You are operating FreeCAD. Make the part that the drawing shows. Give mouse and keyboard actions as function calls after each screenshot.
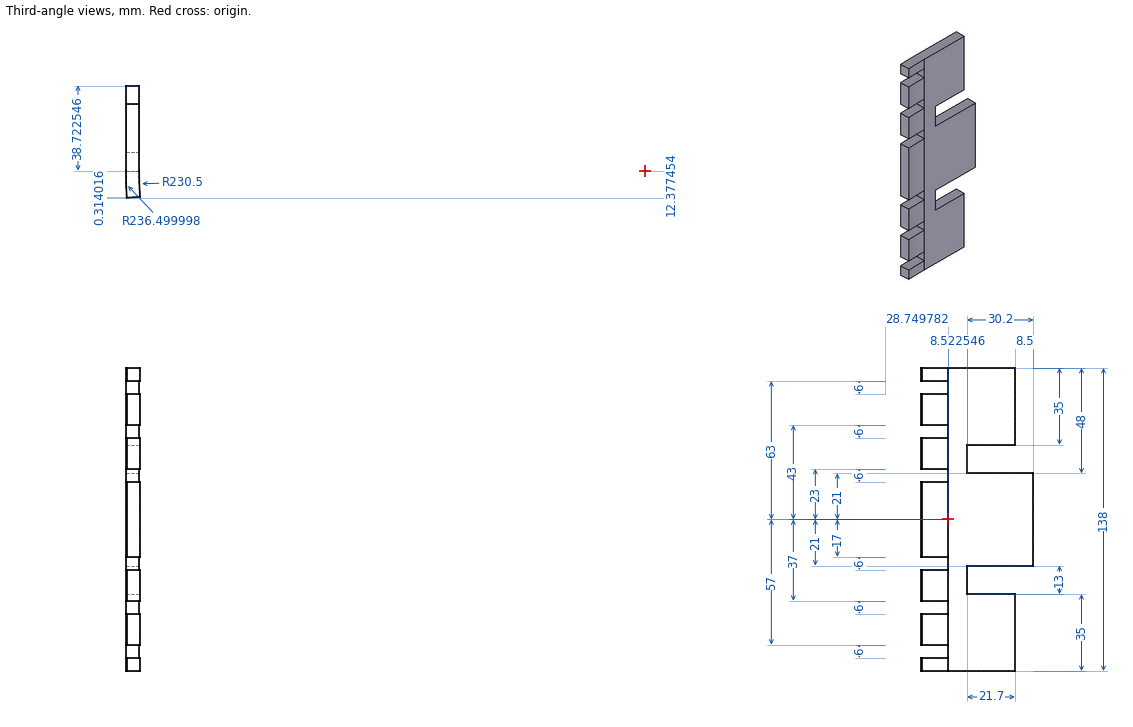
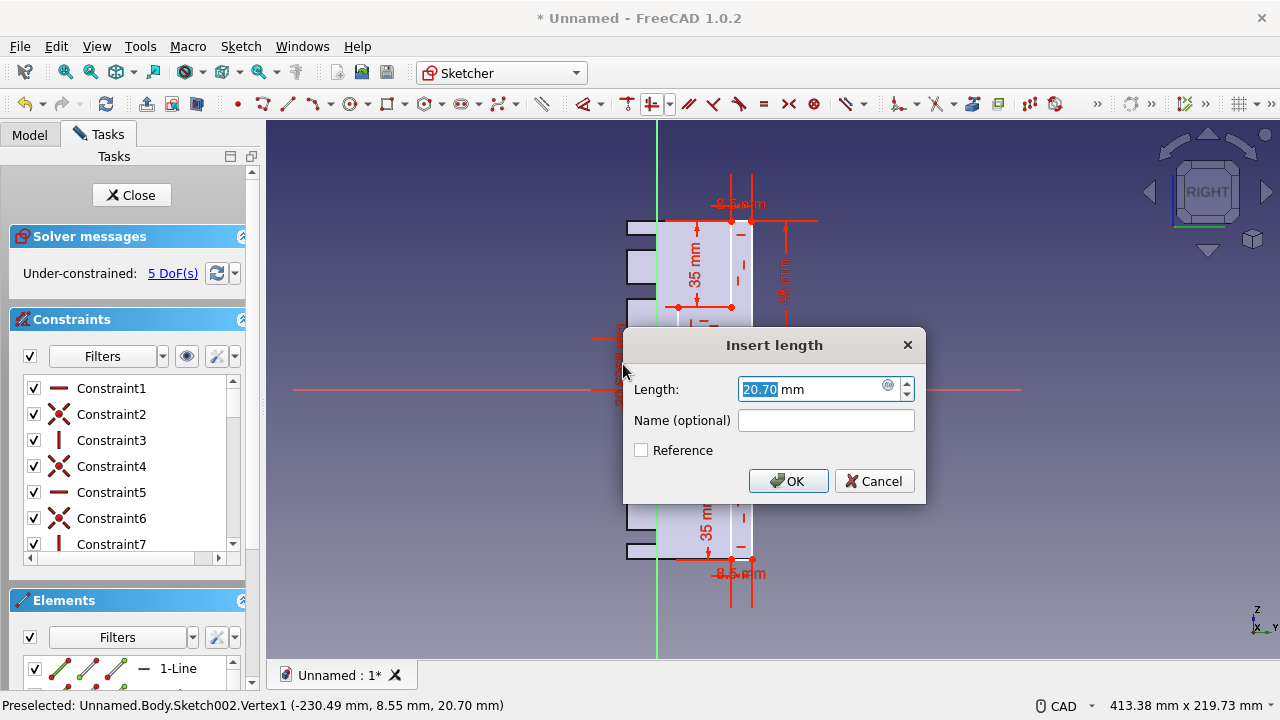
text(21)
key(Return)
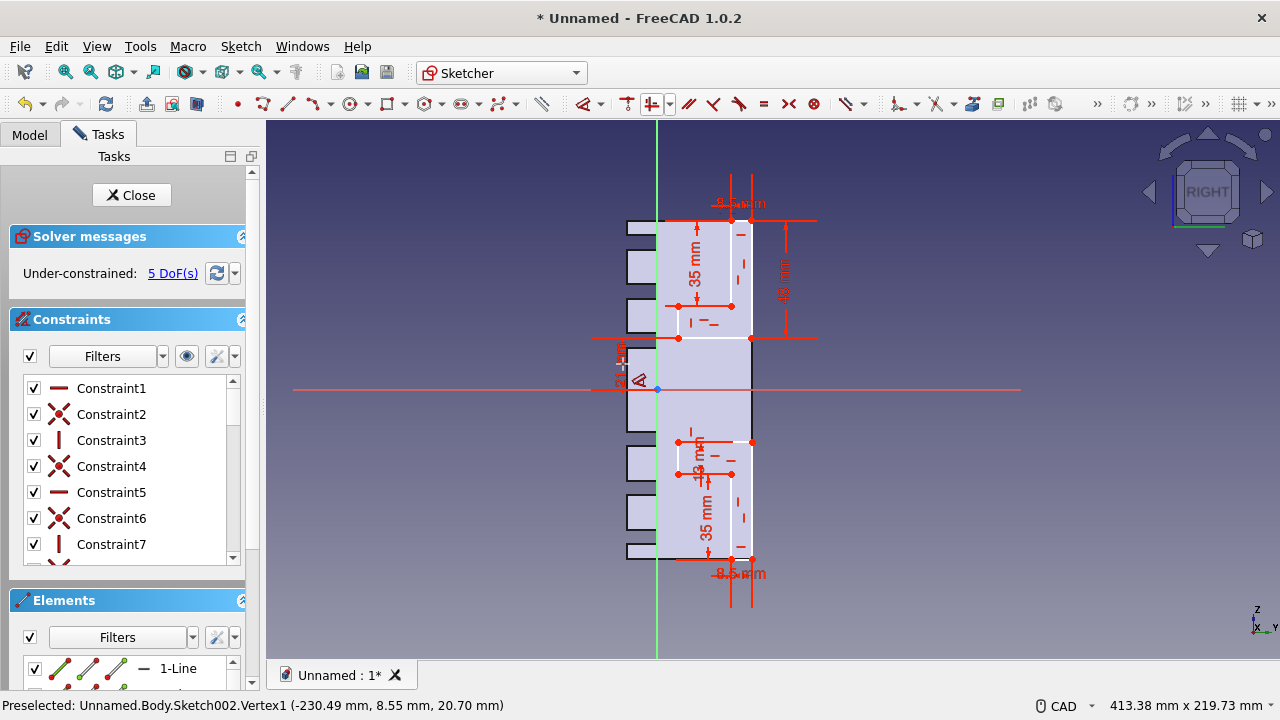
click(678, 442)
click(623, 416)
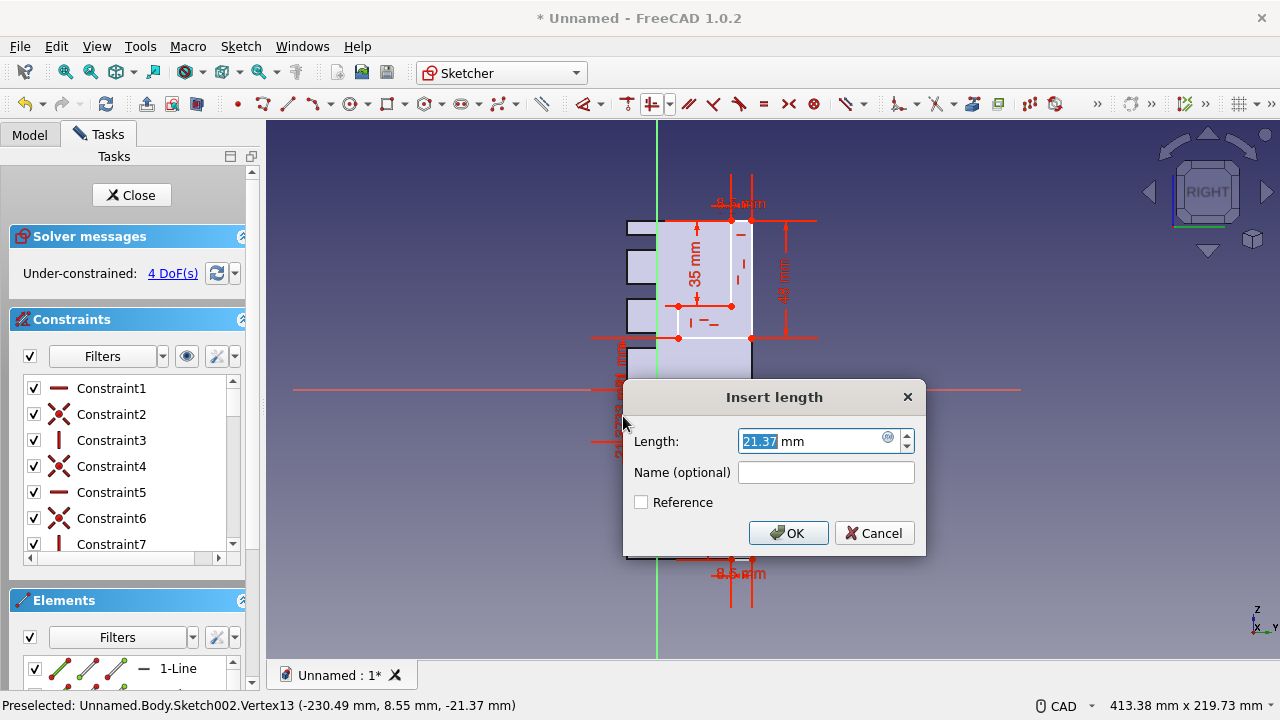
text(21)
key(Return)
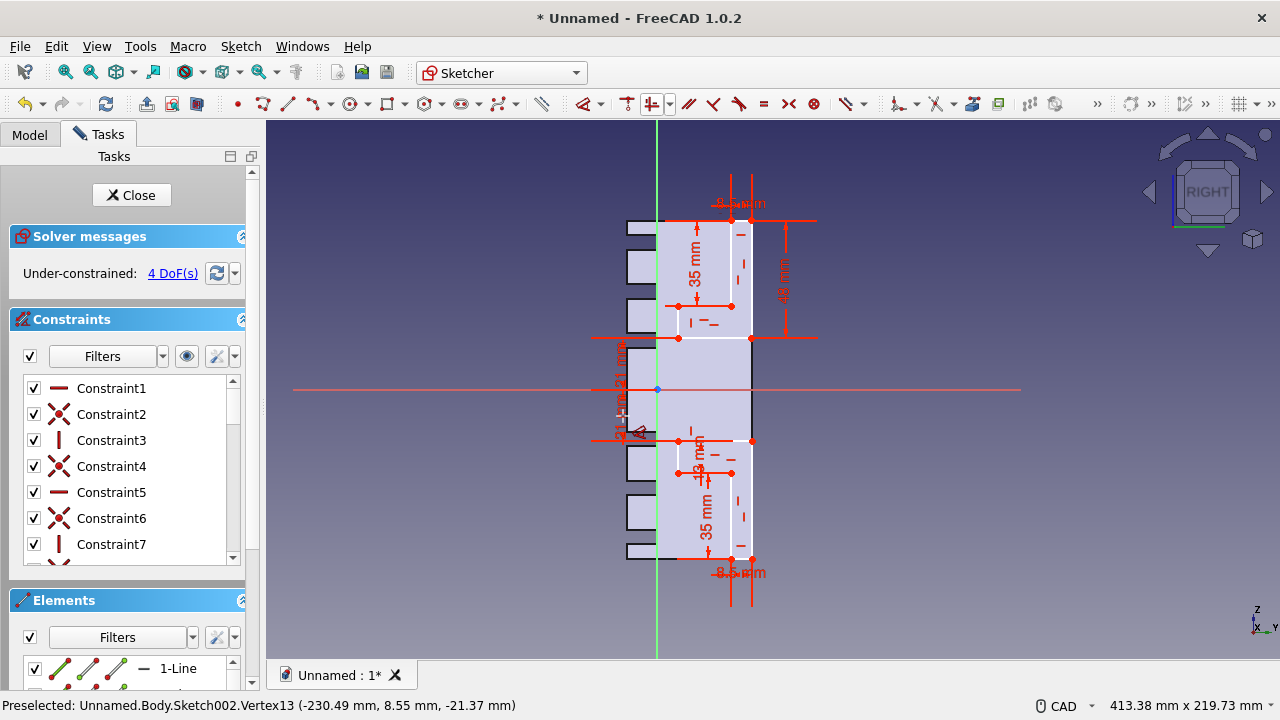
click(700, 338)
click(715, 372)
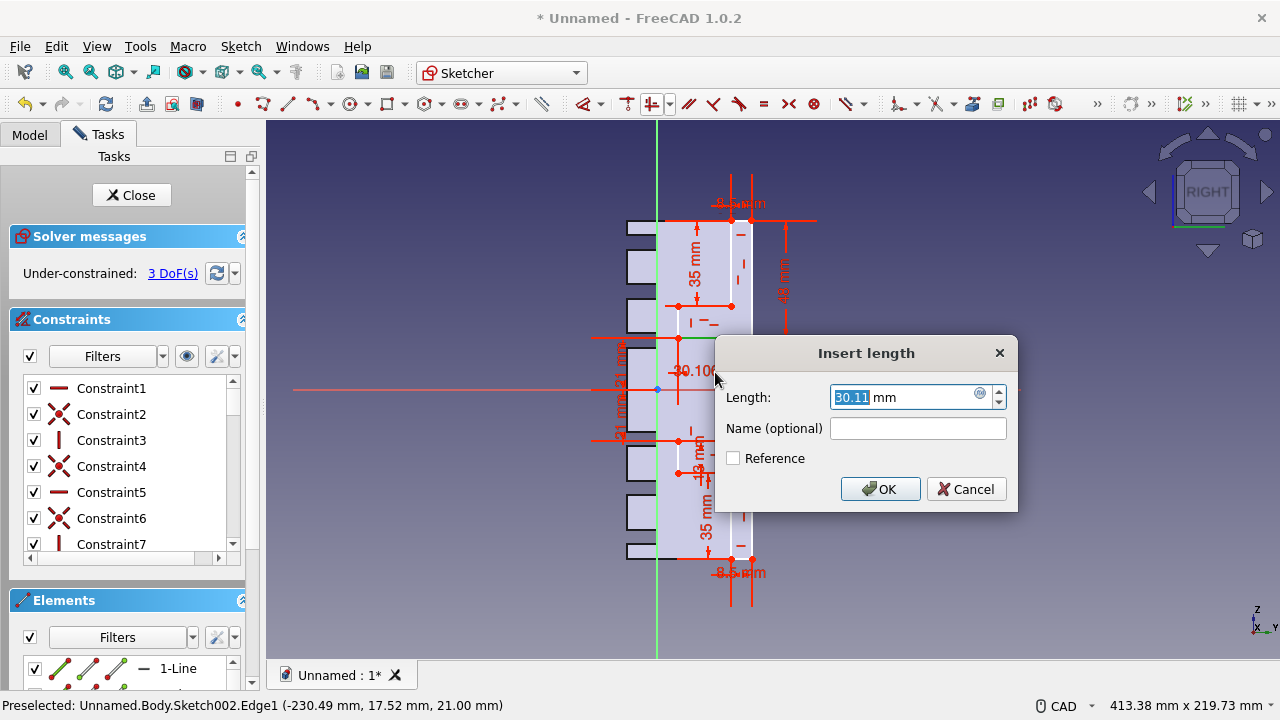
text(30.2)
key(Return)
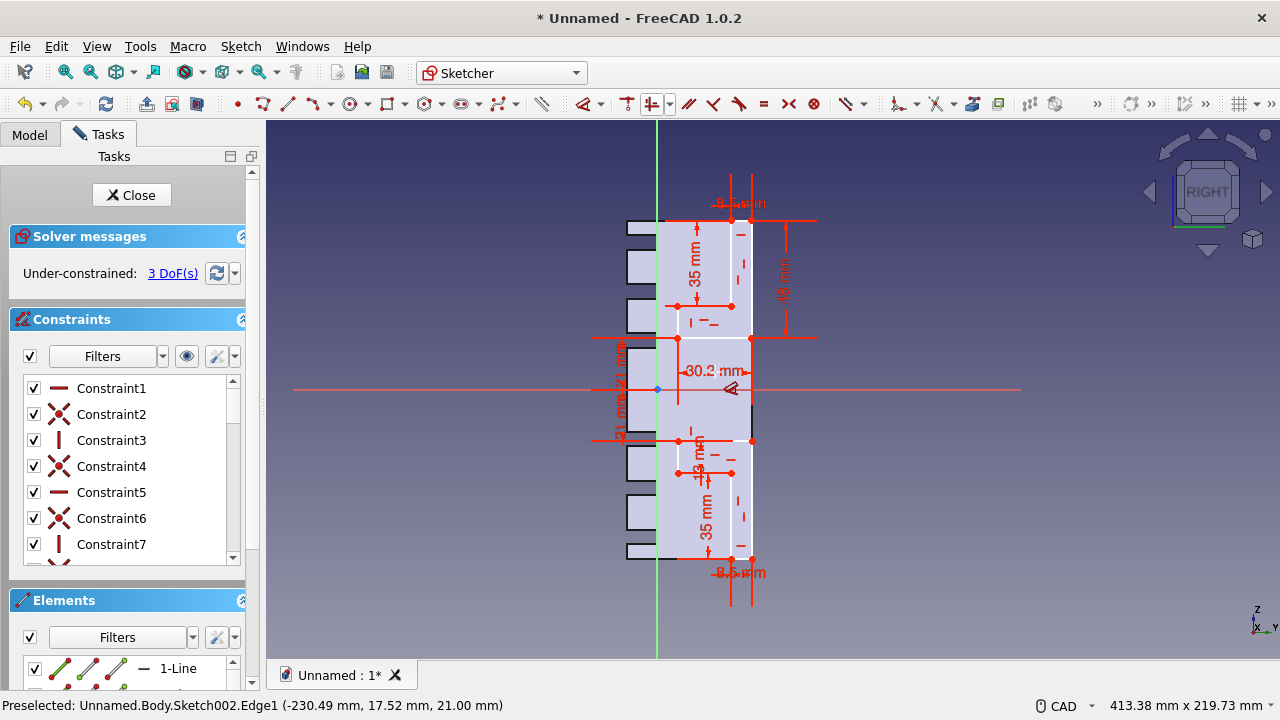
click(694, 473)
click(705, 415)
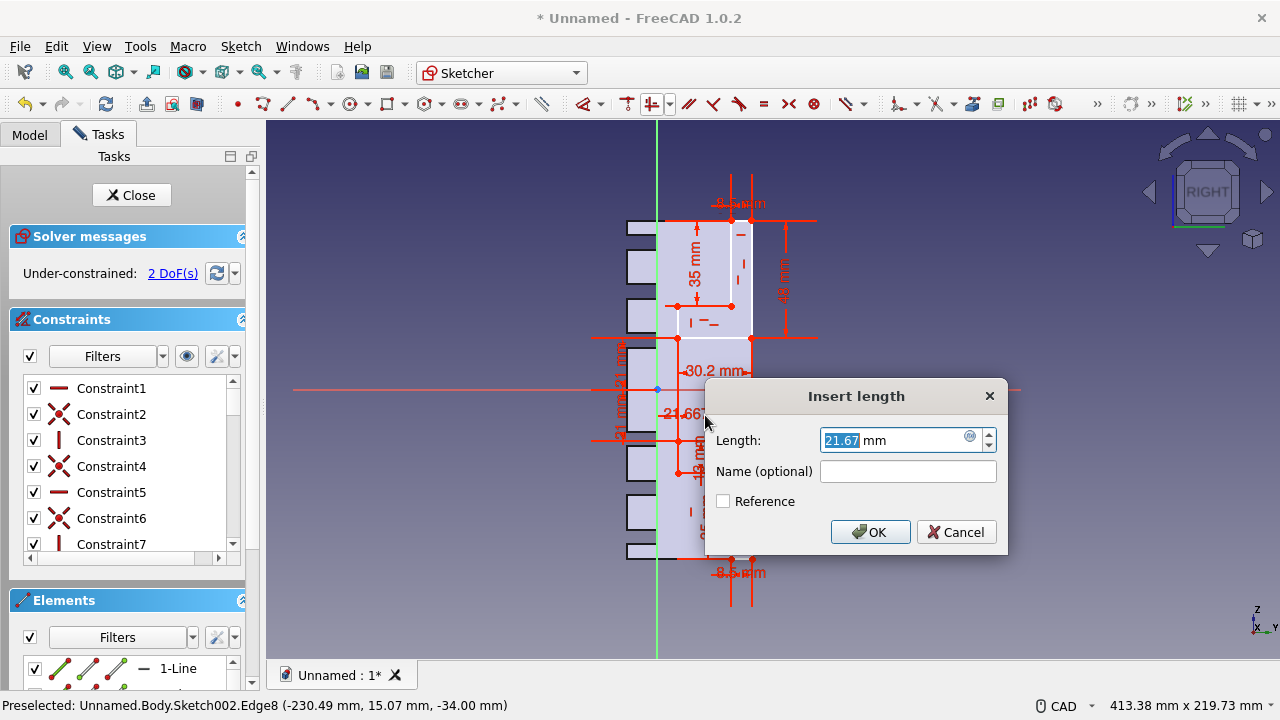
text(21.7)
key(Return)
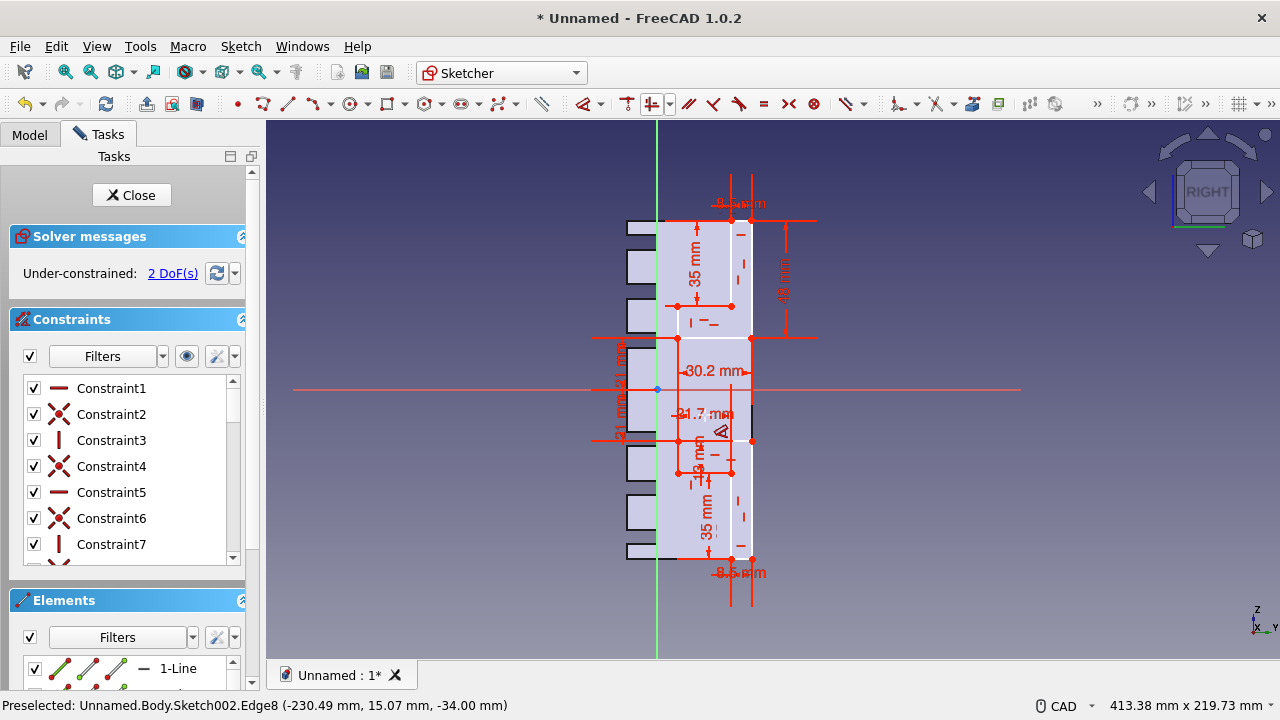
scroll(678, 338, up, 4)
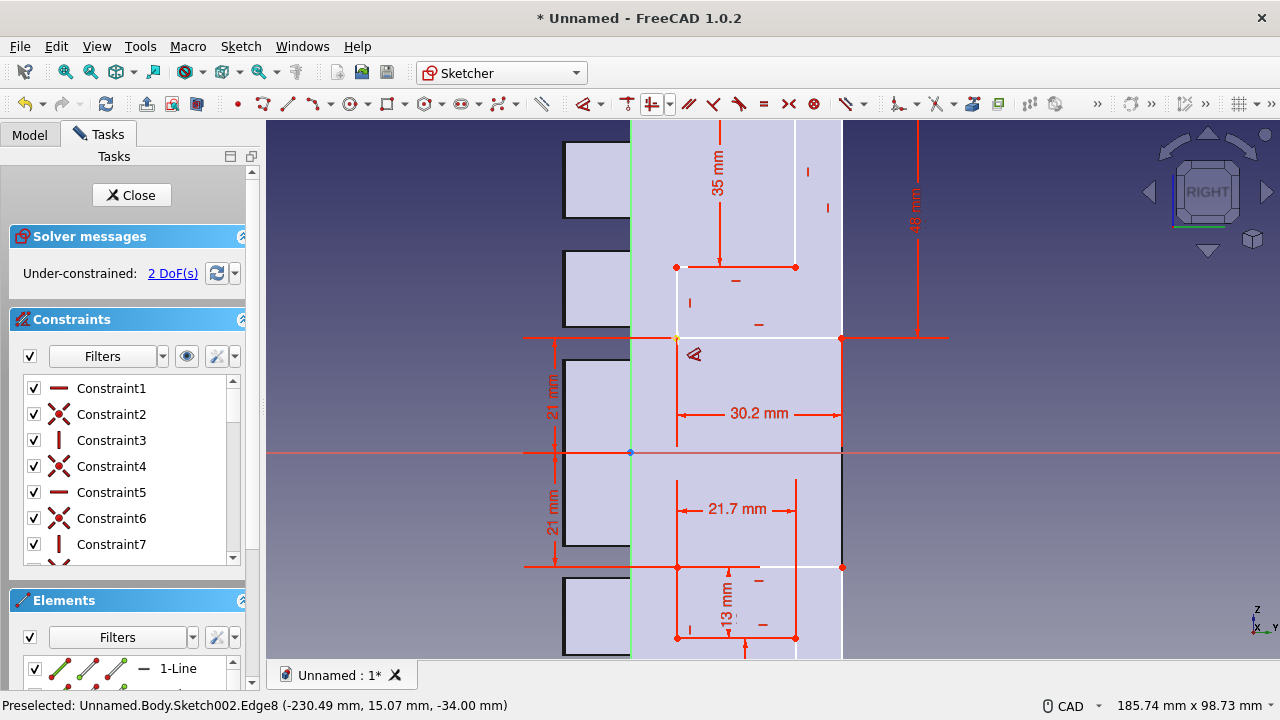
click(677, 338)
click(654, 304)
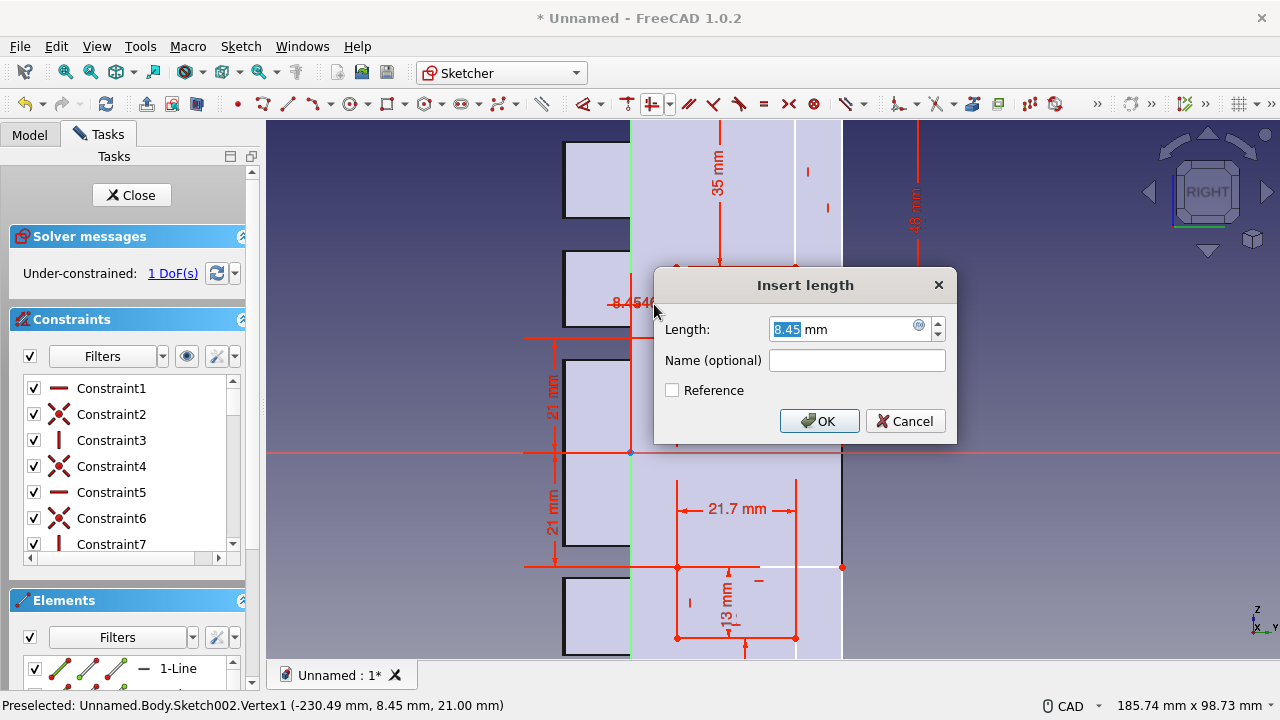
text(8.522546)
key(Return)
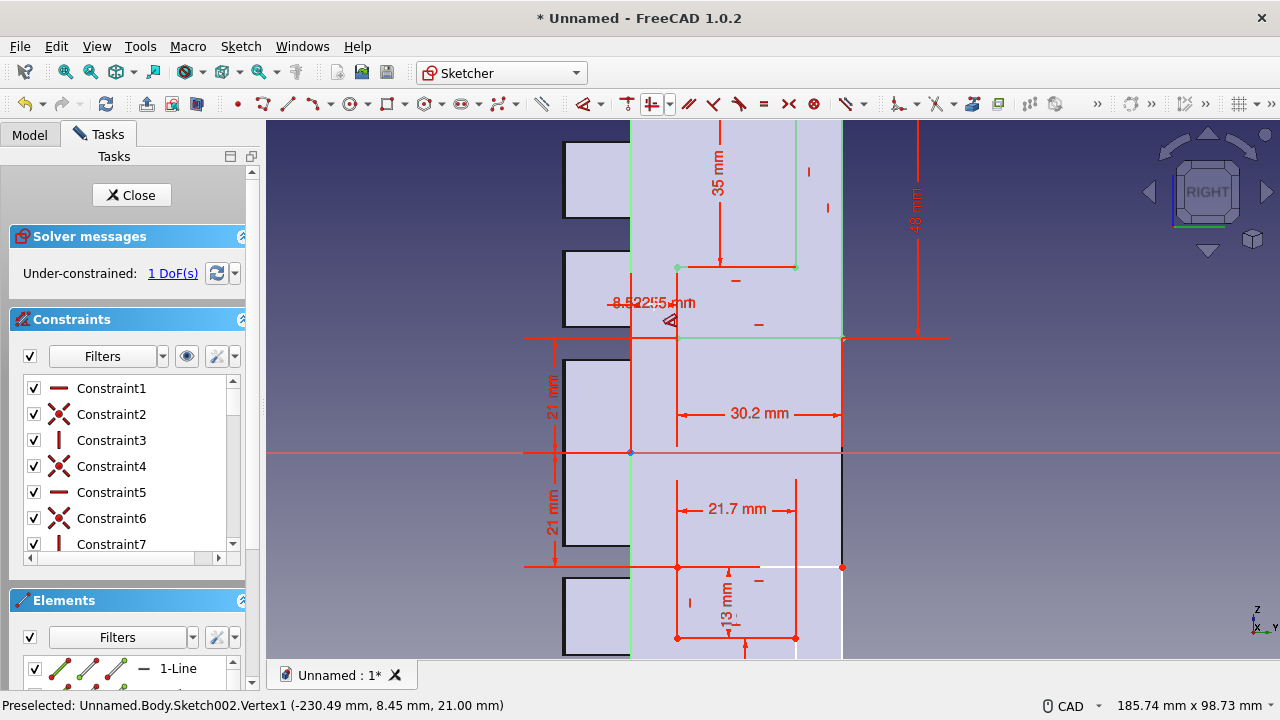
click(678, 567)
click(654, 601)